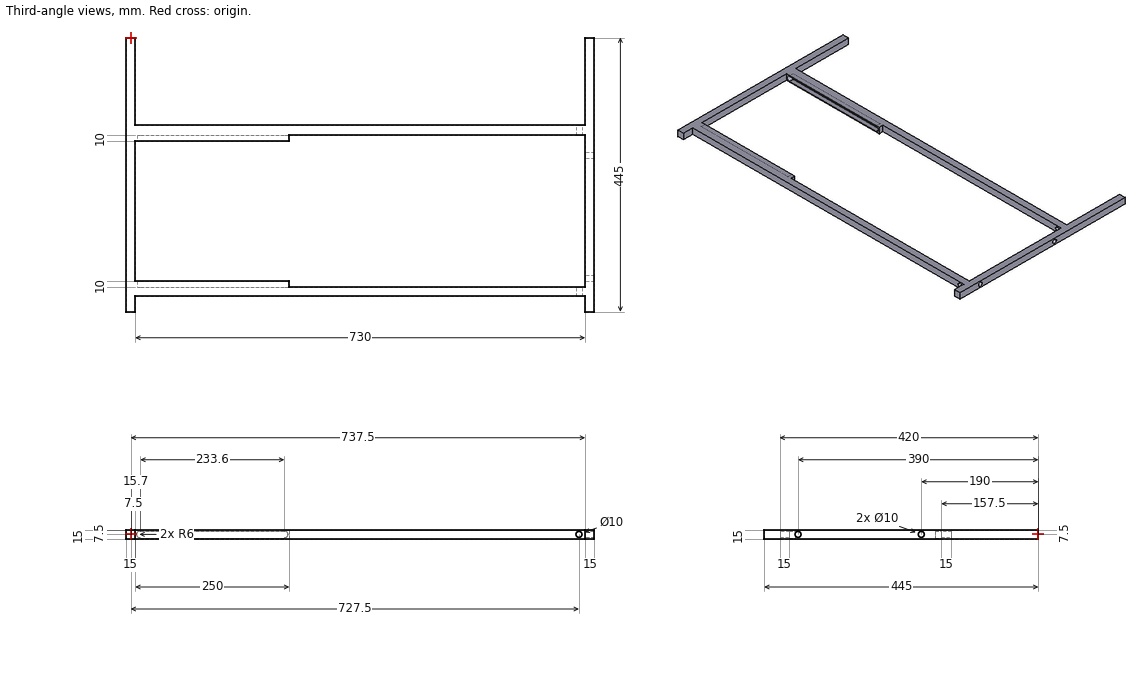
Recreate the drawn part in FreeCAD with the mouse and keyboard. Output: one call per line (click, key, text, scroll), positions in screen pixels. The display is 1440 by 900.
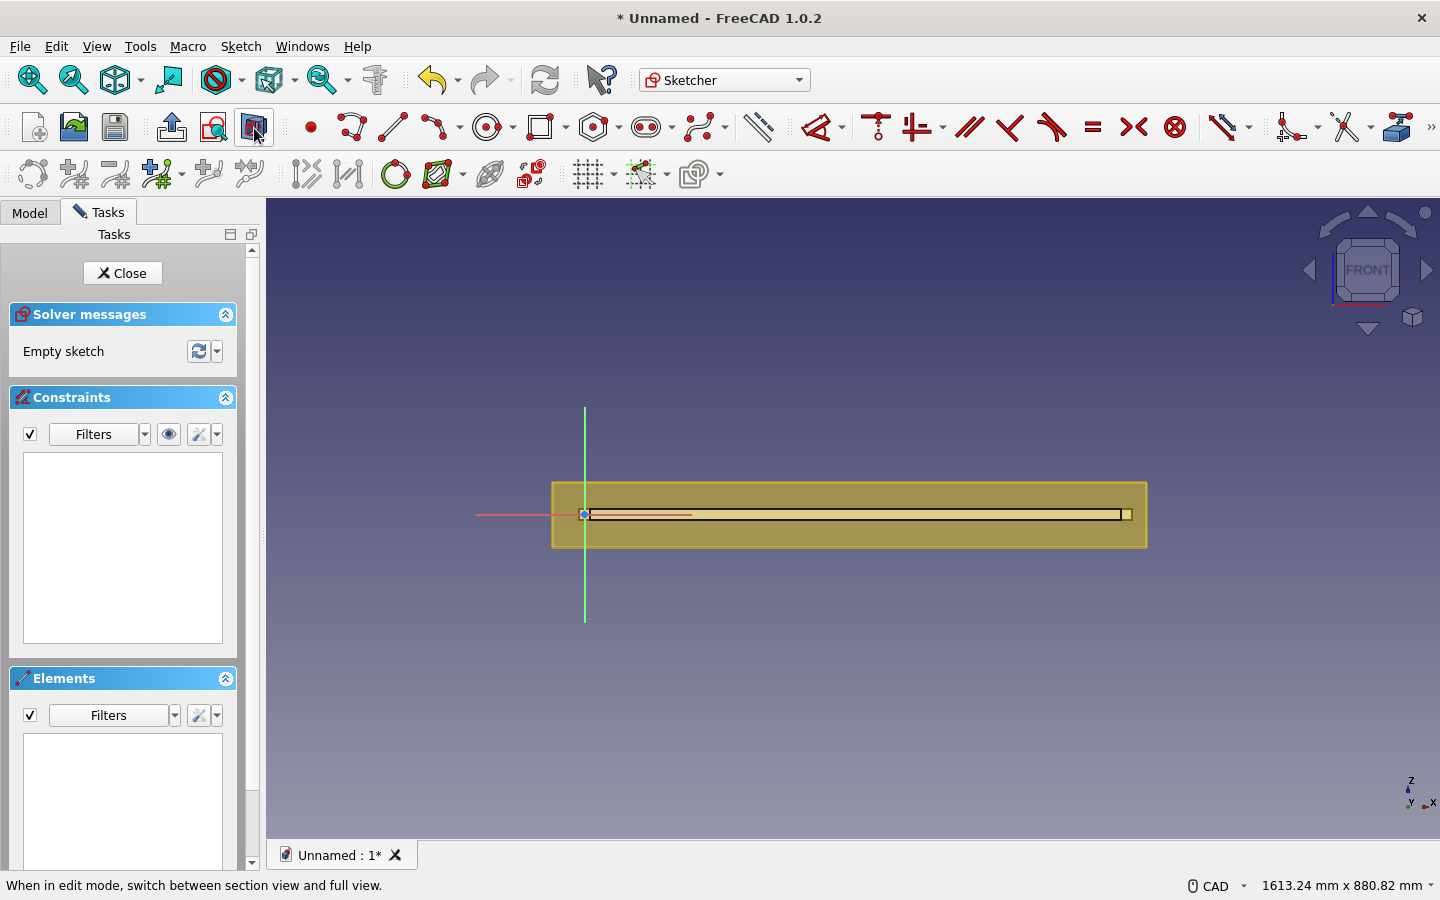
scroll(644, 513, up, 7)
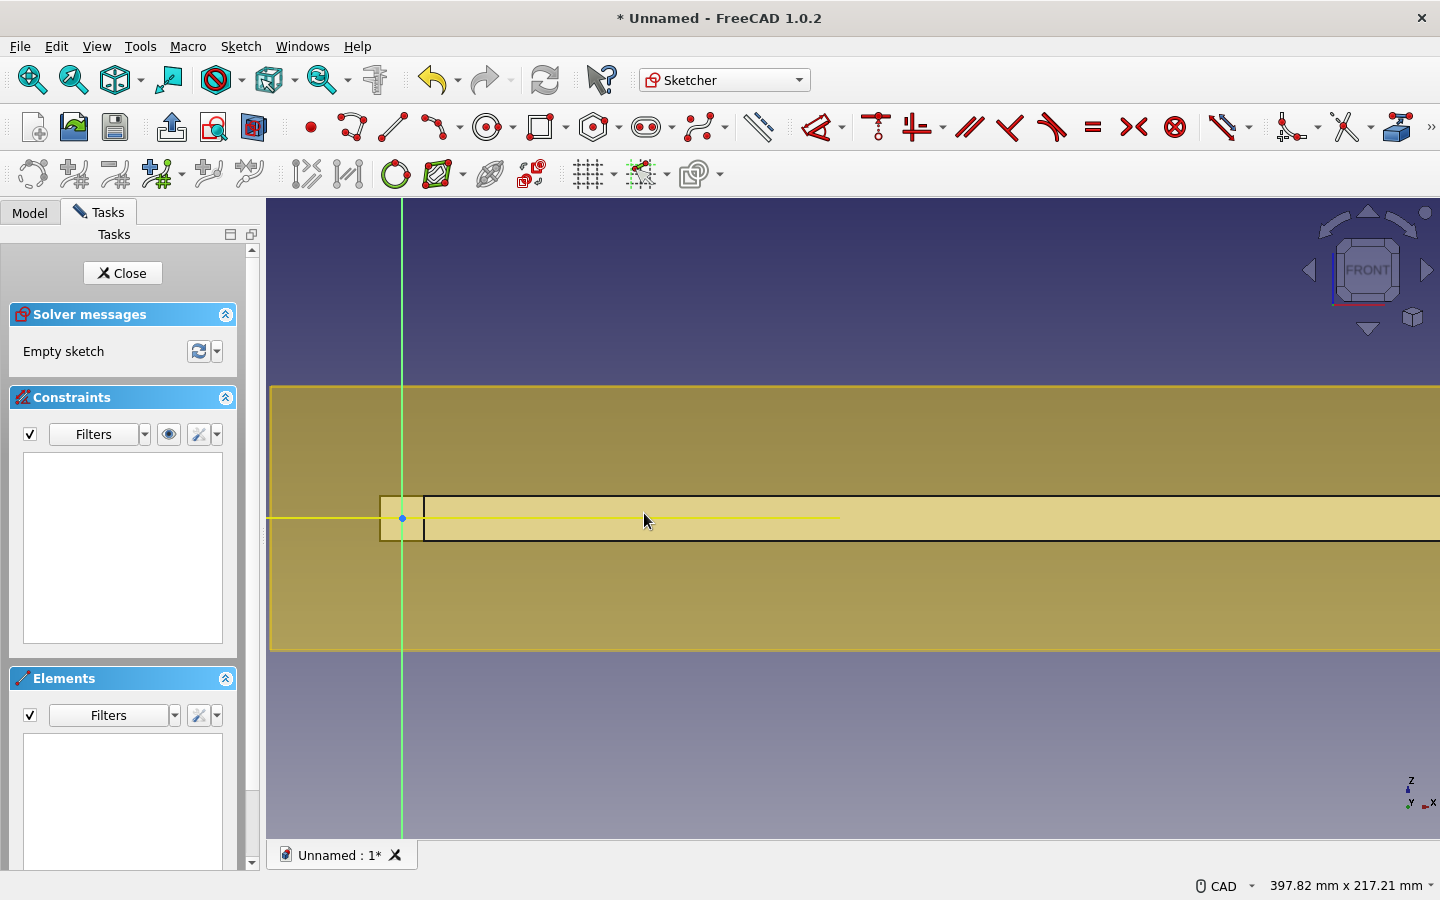
click(540, 128)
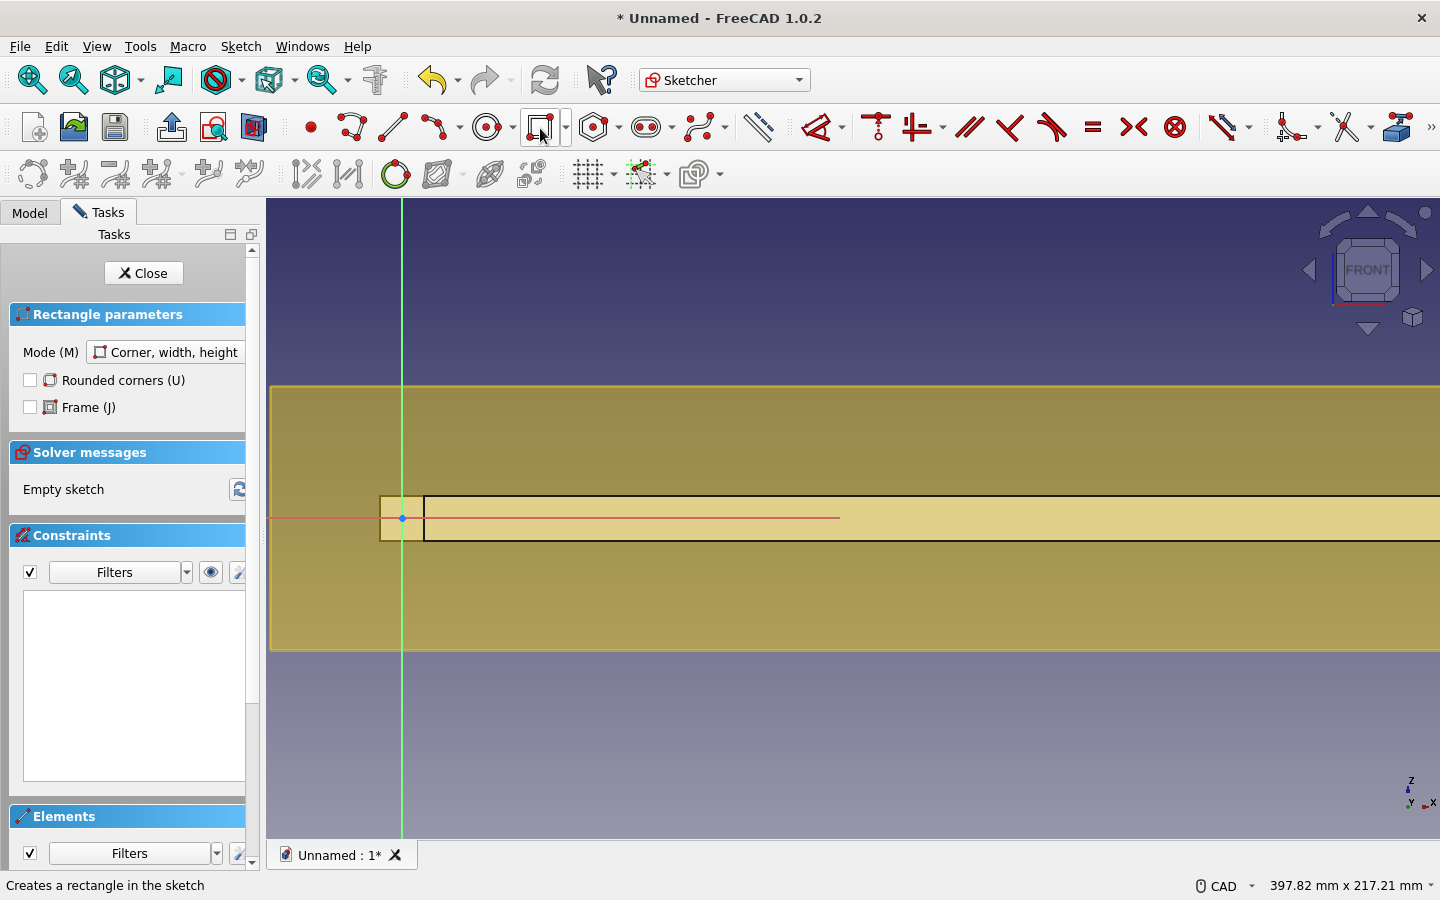
click(424, 496)
click(1162, 541)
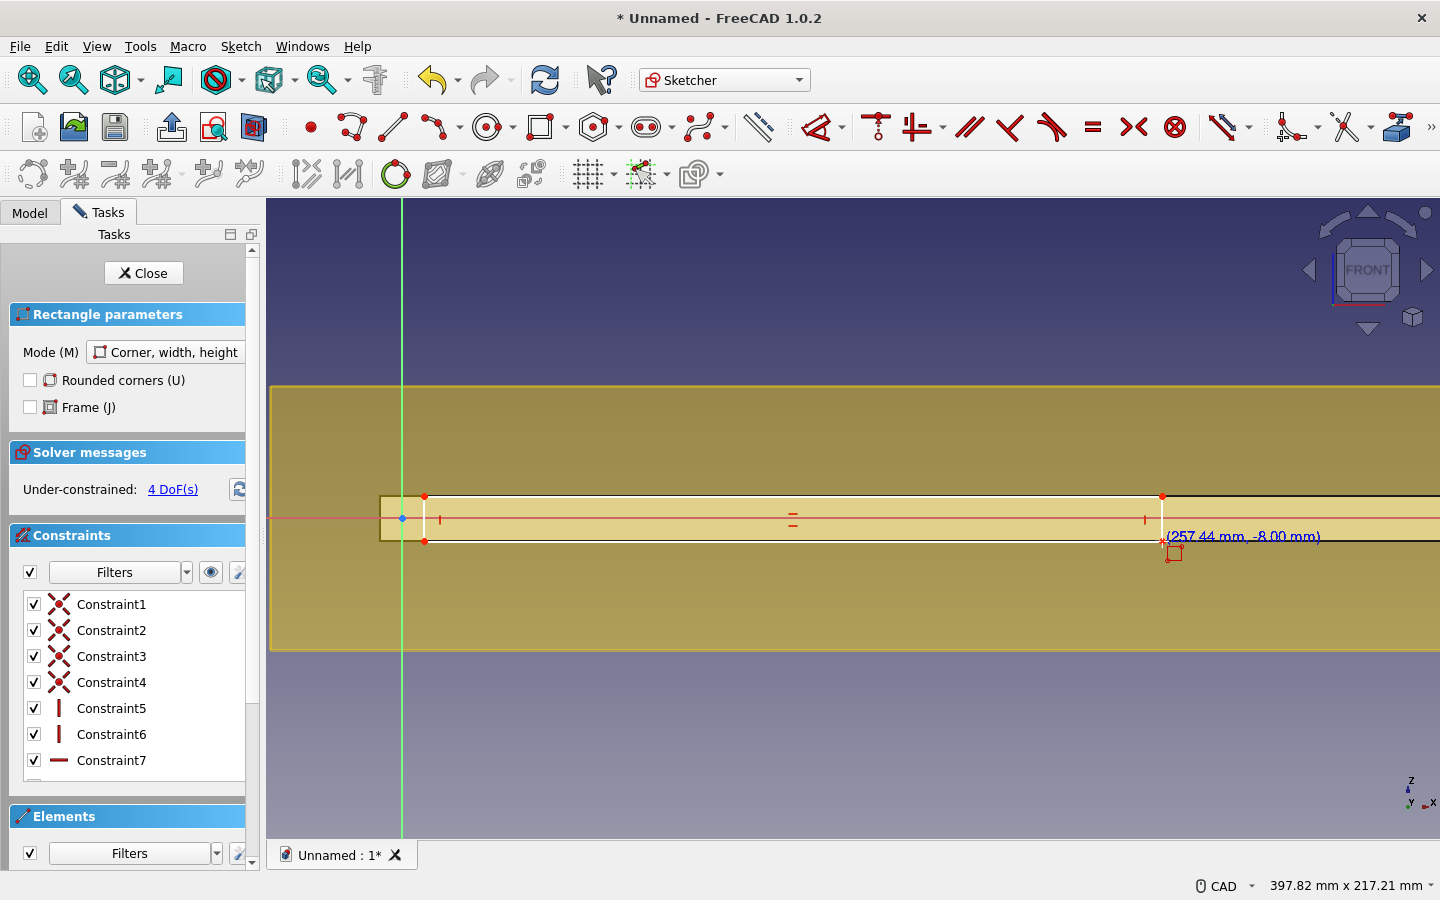
click(646, 128)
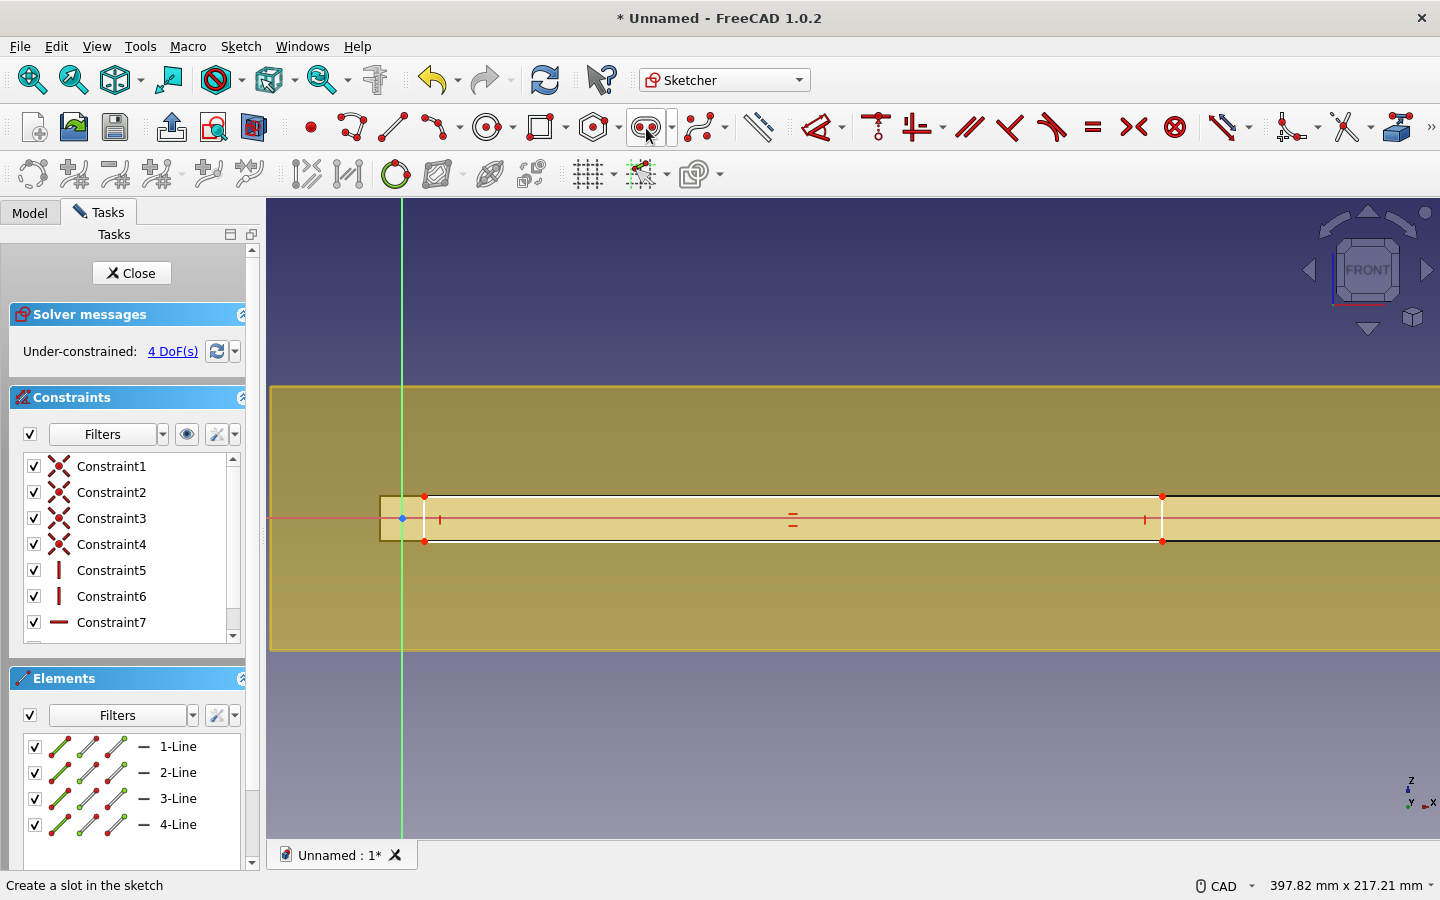
scroll(449, 518, up, 2)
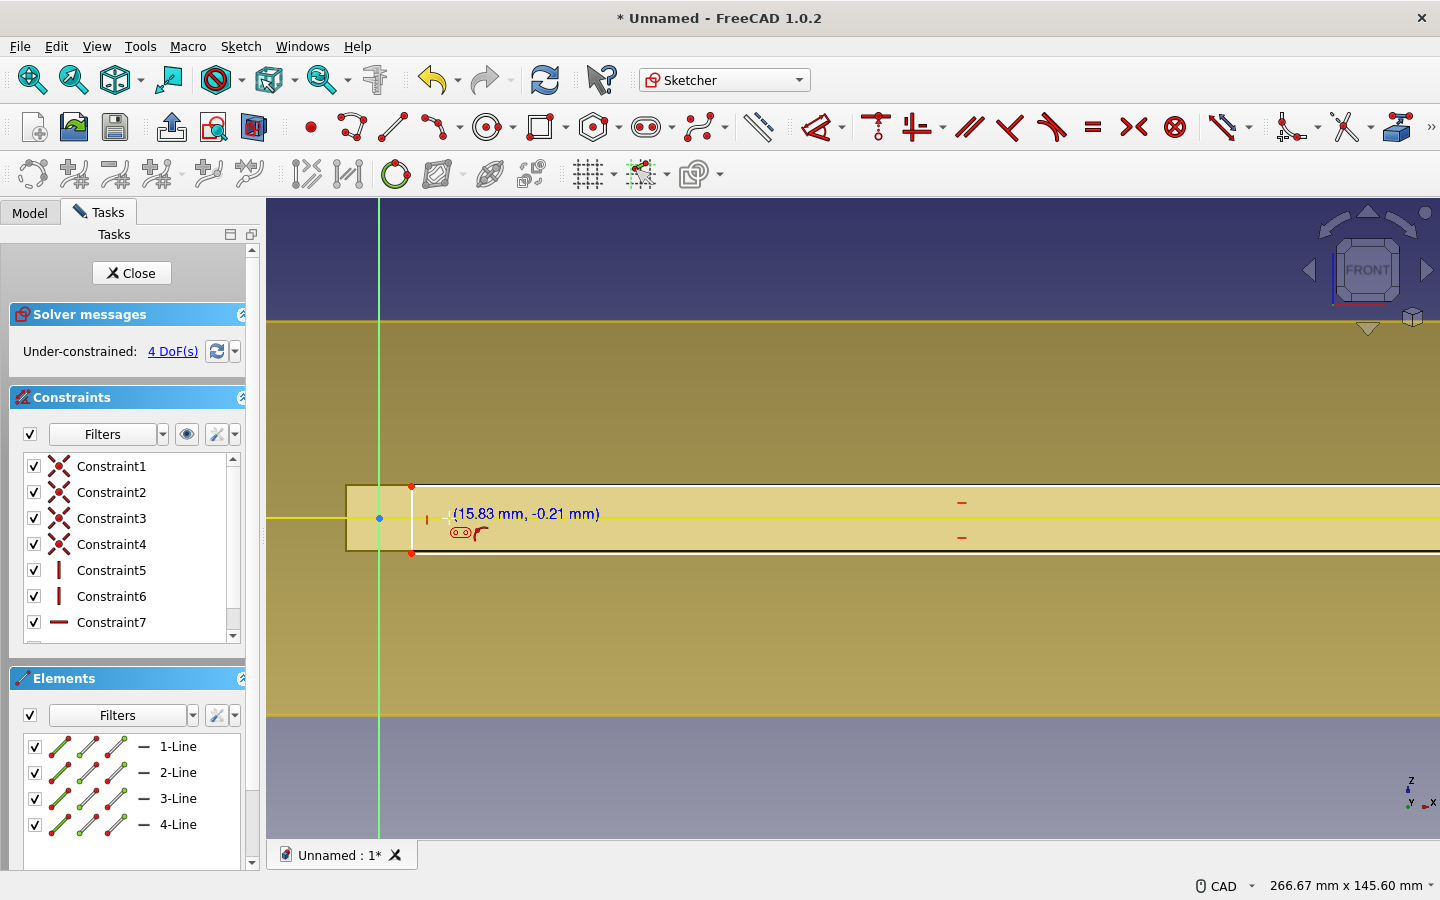
click(448, 518)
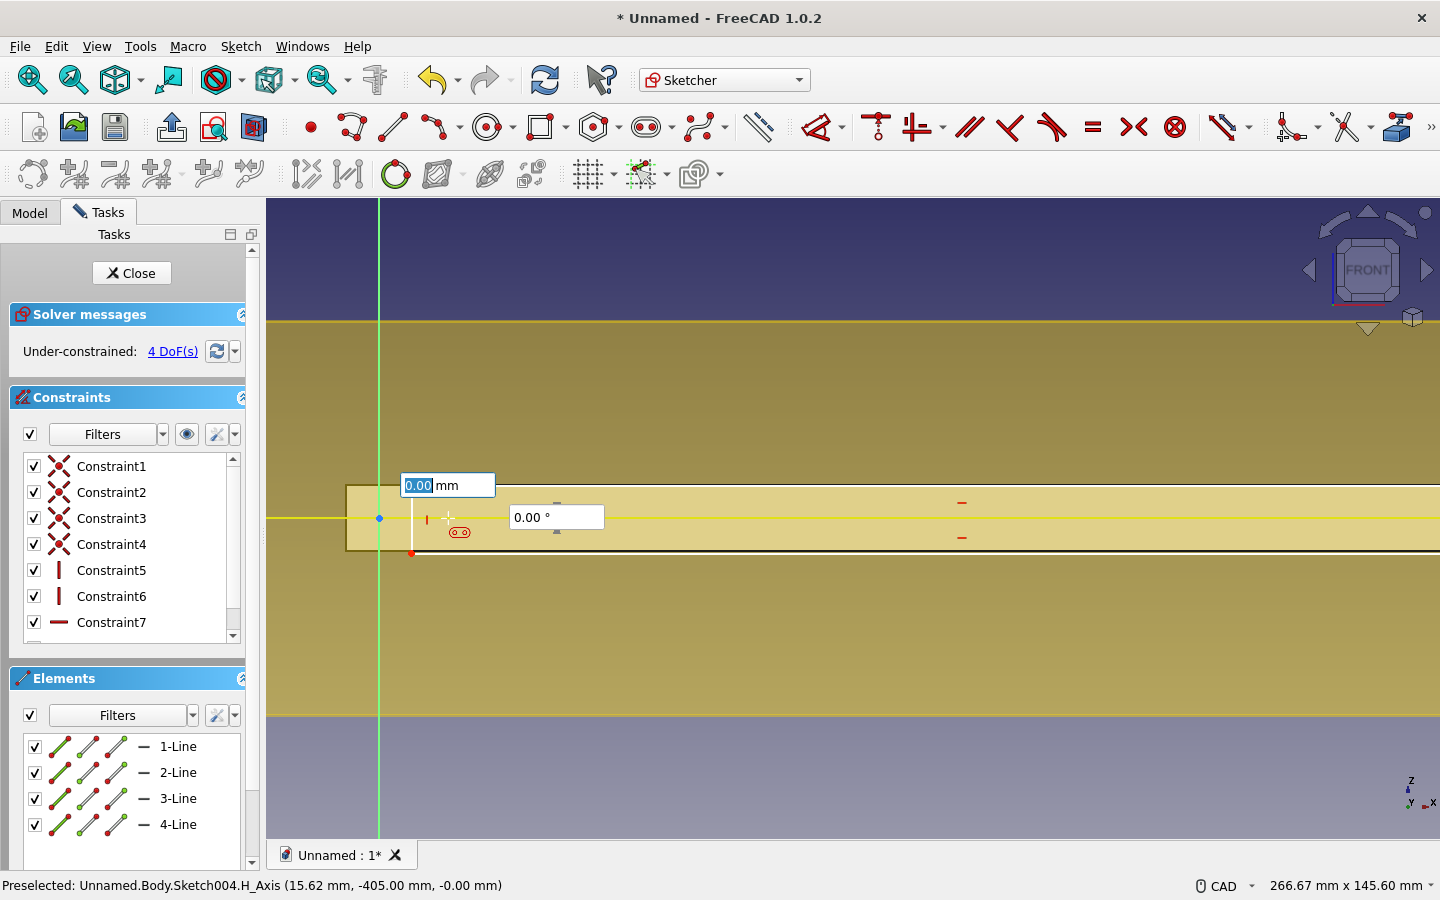
scroll(456, 519, down, 2)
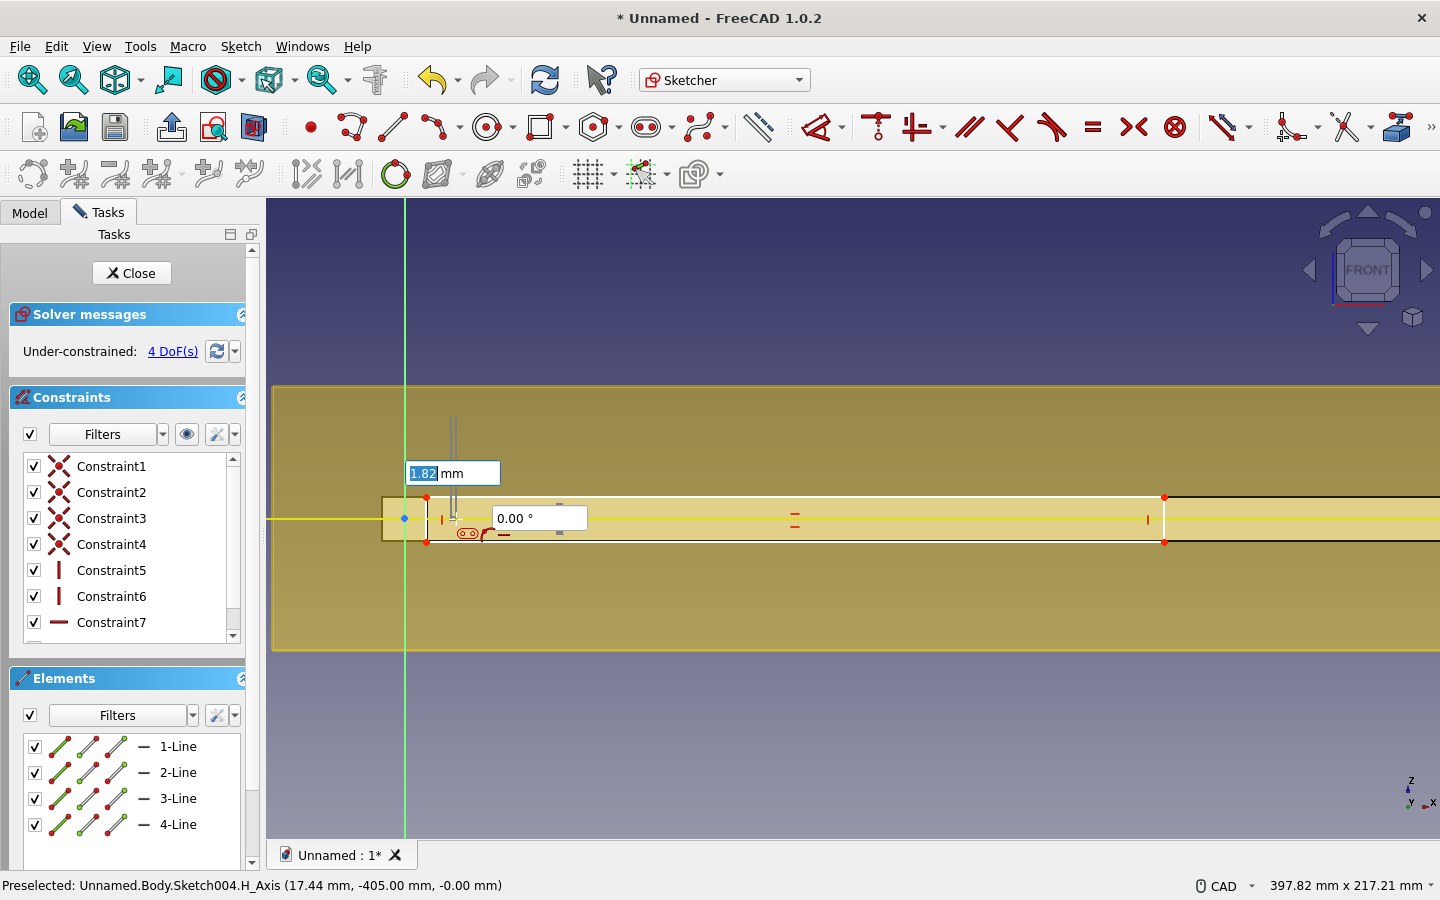
click(1140, 510)